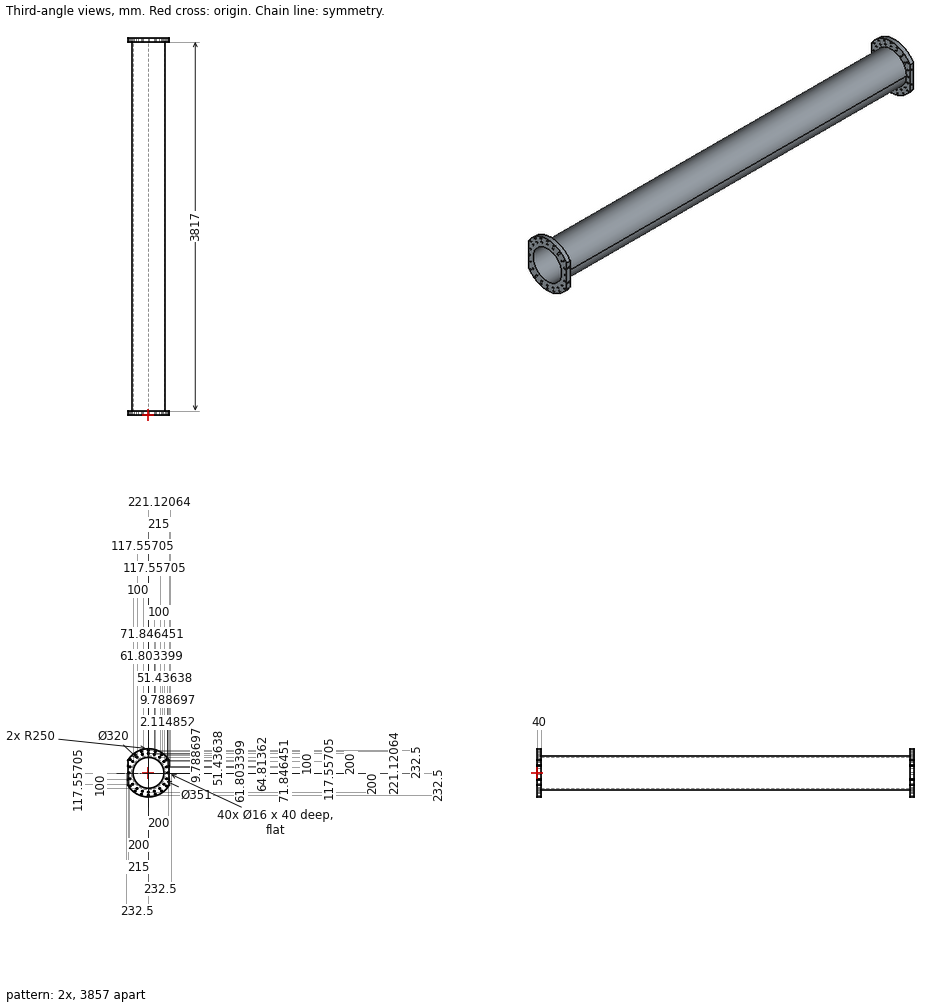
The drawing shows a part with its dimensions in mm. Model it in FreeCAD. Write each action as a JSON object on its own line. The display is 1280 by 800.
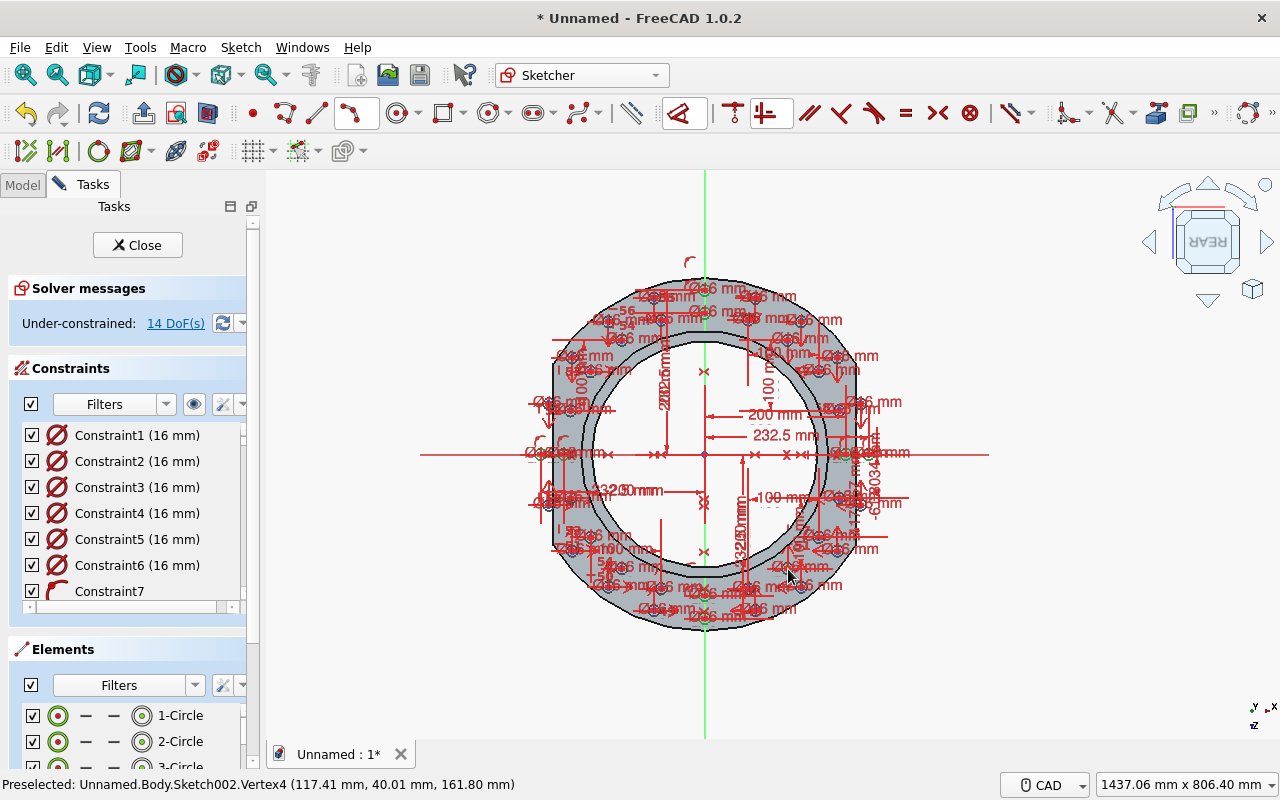
{"action": "key", "text": "l"}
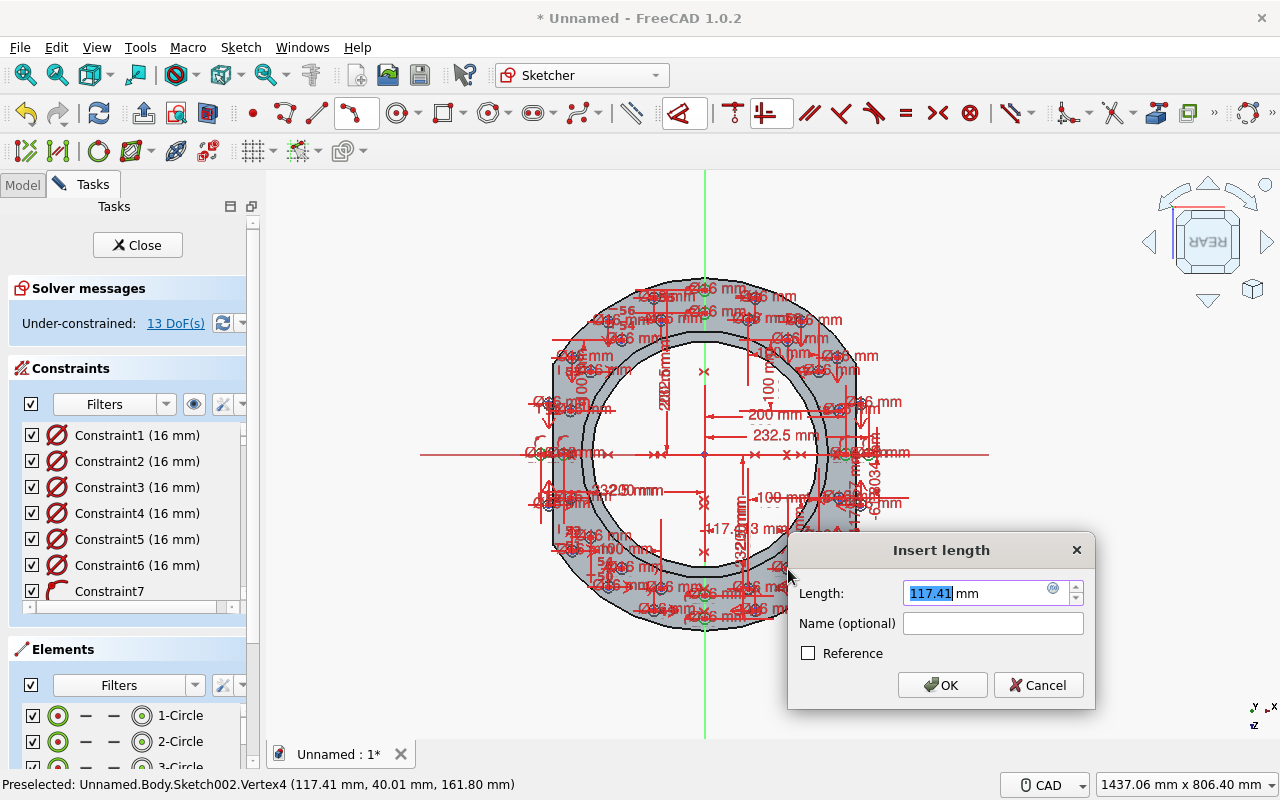
{"action": "type", "text": "117.55705"}
{"action": "key", "text": "Return"}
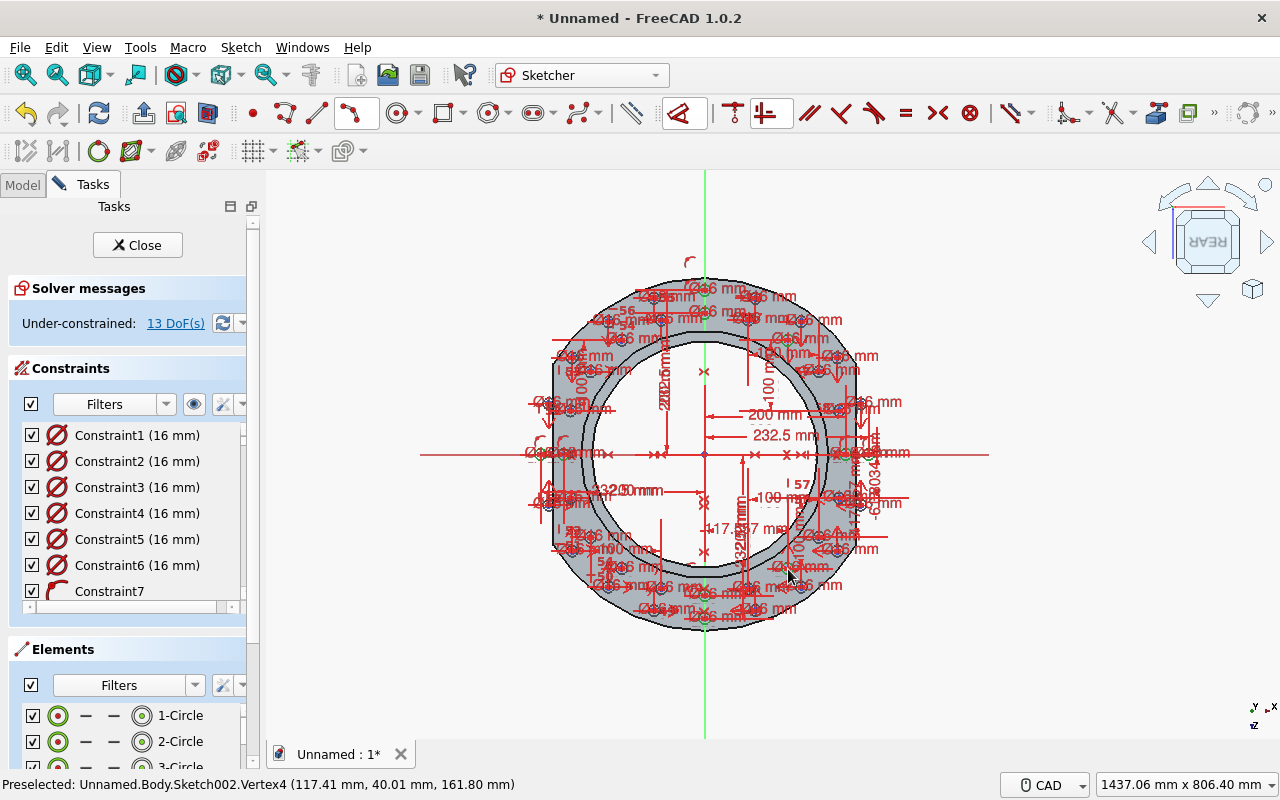
{"action": "left_click", "coordinate": [748, 589]}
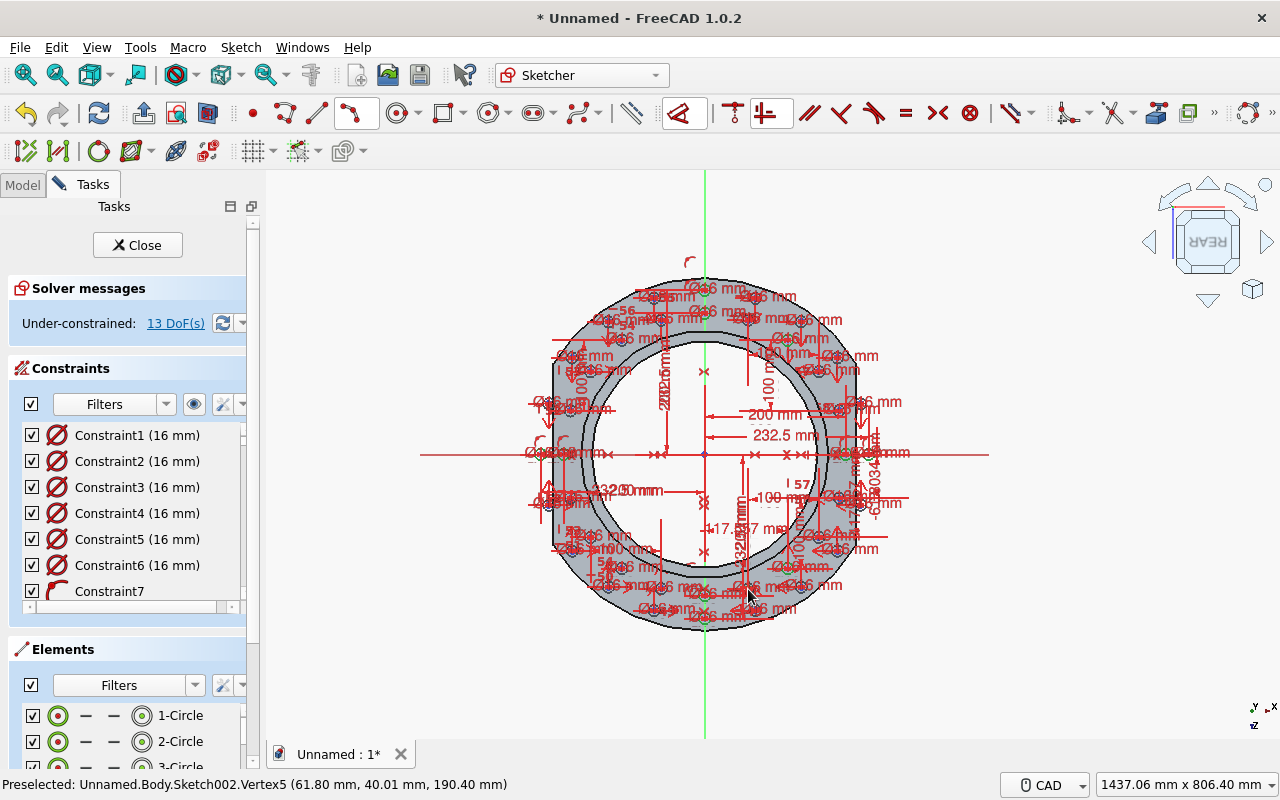
{"action": "key", "text": "l"}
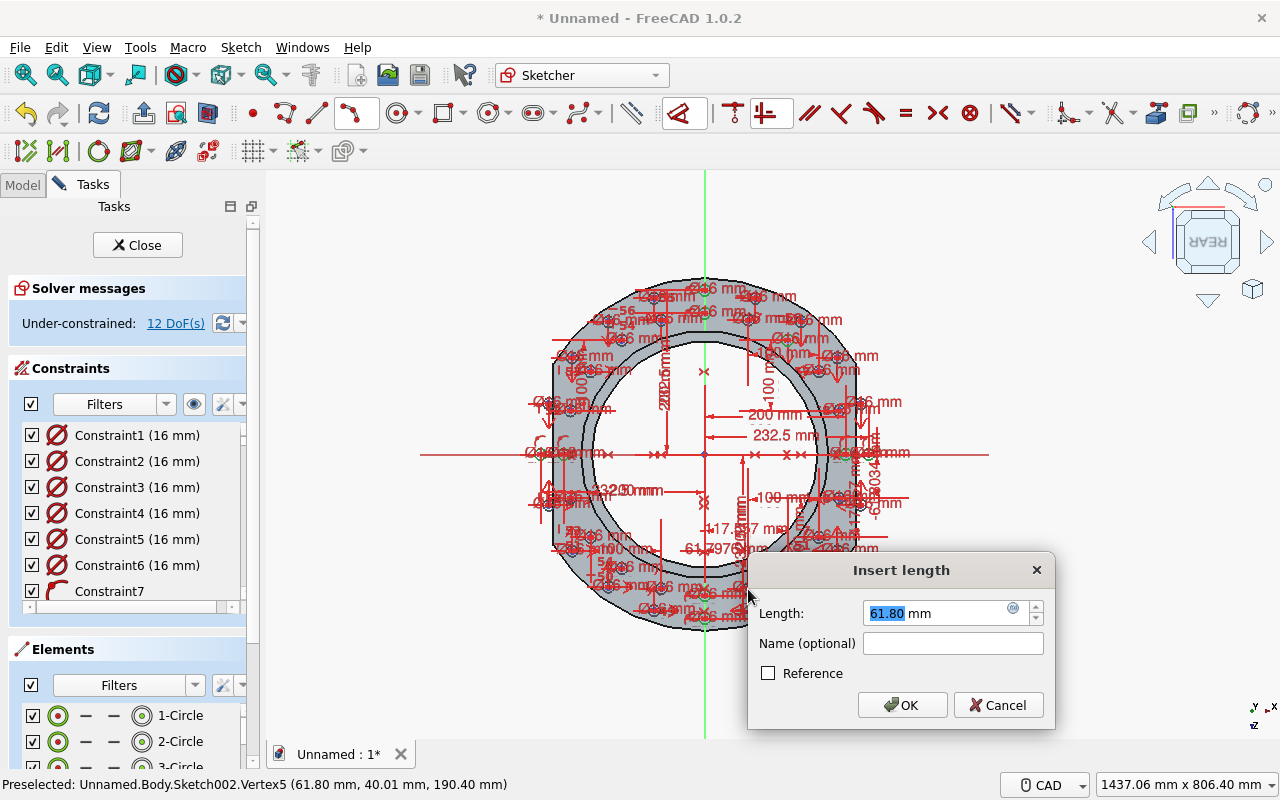
{"action": "type", "text": "61.803399"}
{"action": "key", "text": "Return"}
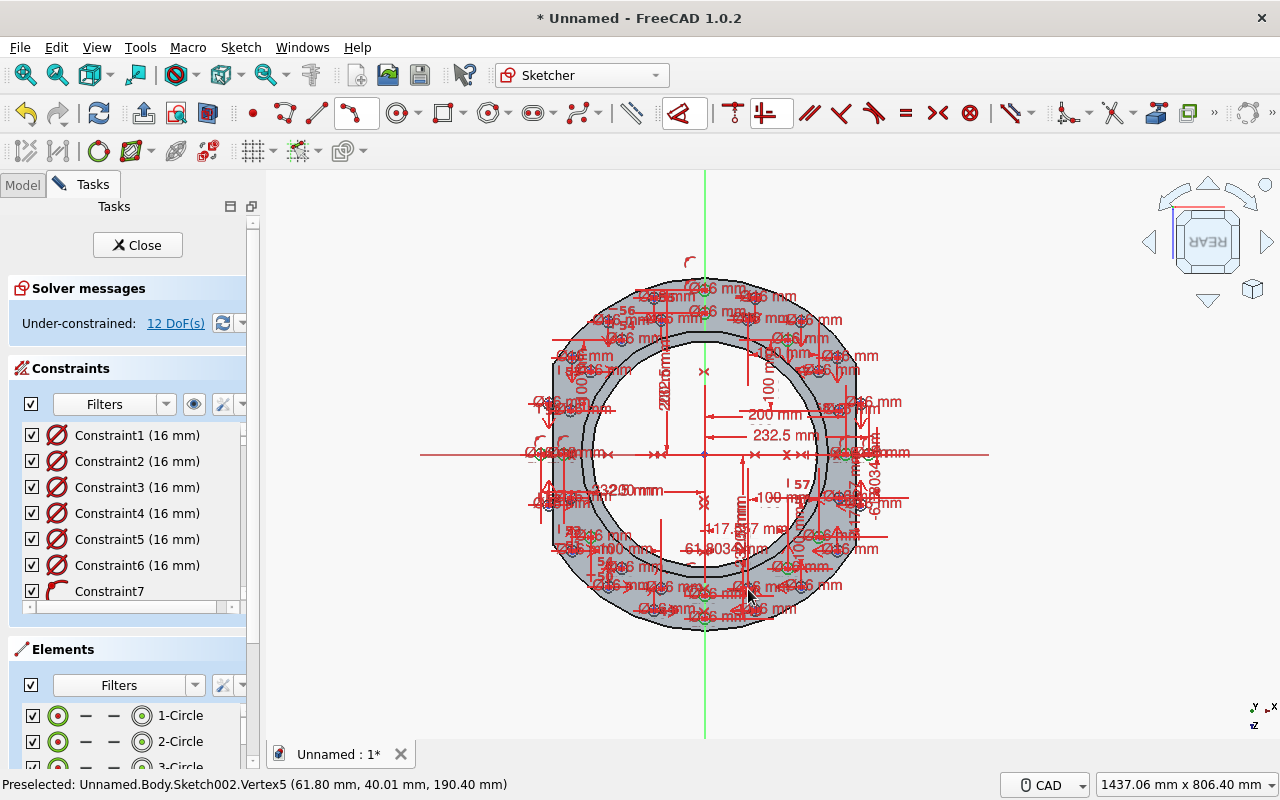
{"action": "left_click", "coordinate": [622, 569]}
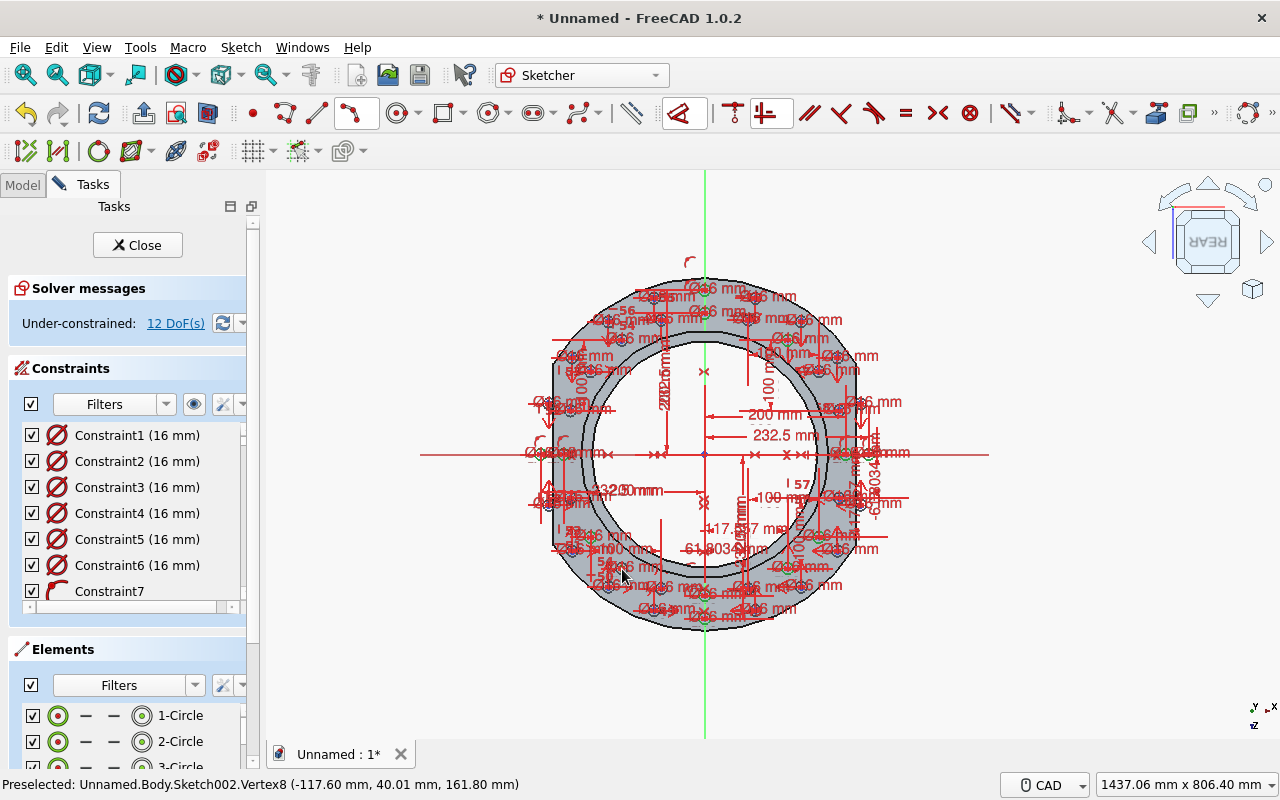
{"action": "key", "text": "l"}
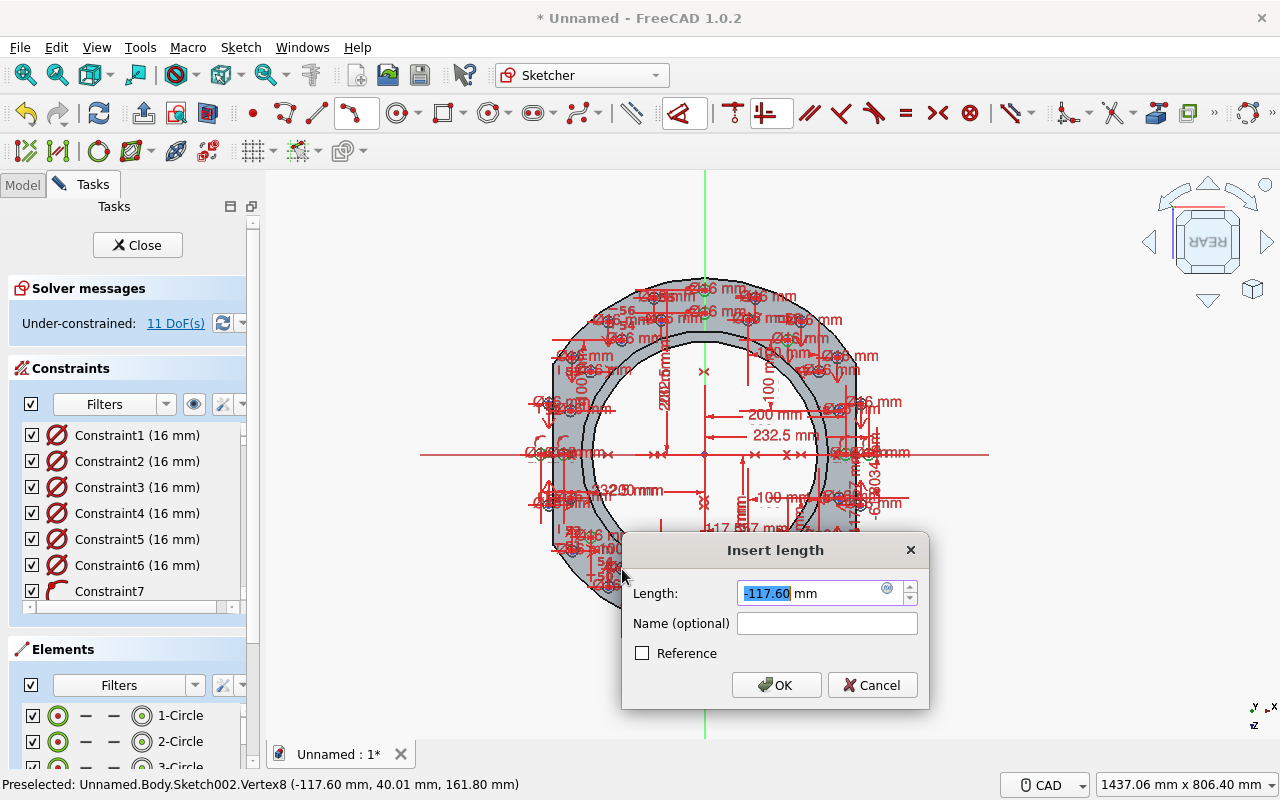
{"action": "type", "text": "-117.55705"}
{"action": "key", "text": "Return"}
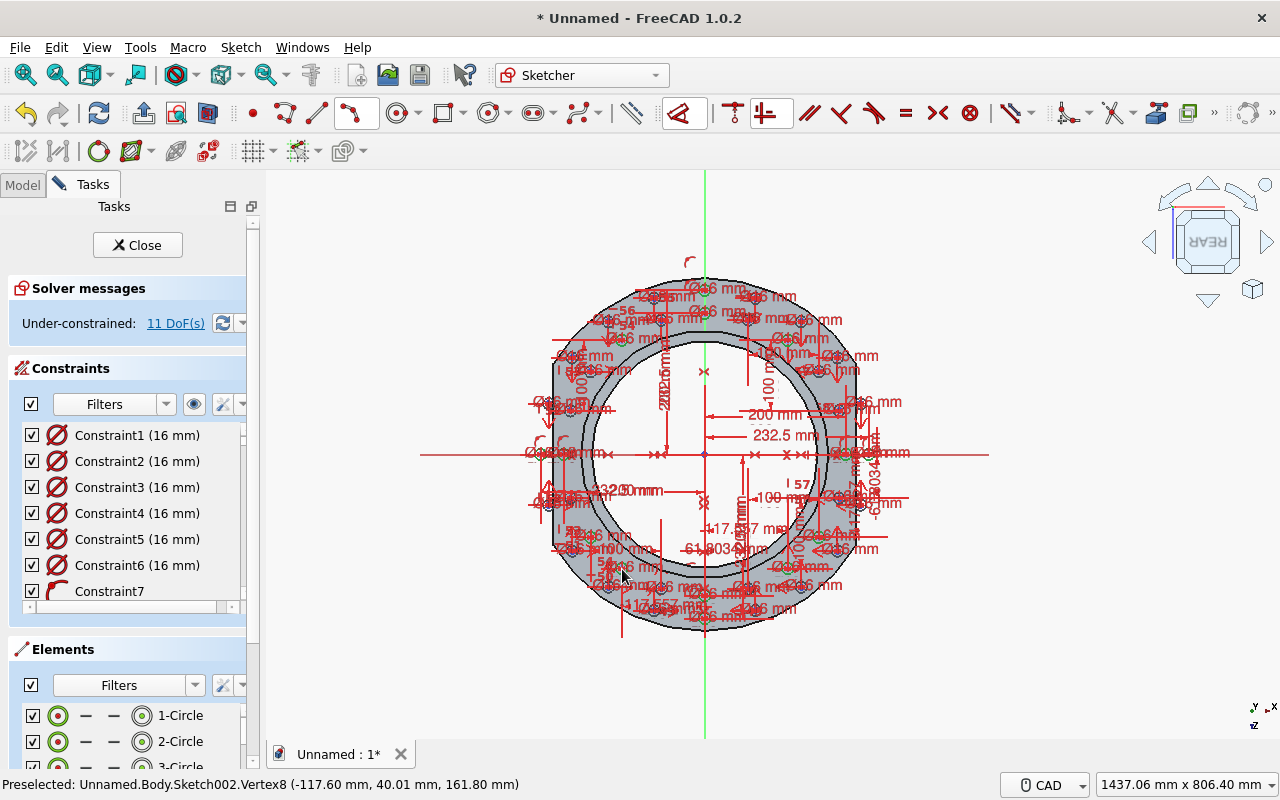
{"action": "left_click", "coordinate": [591, 372]}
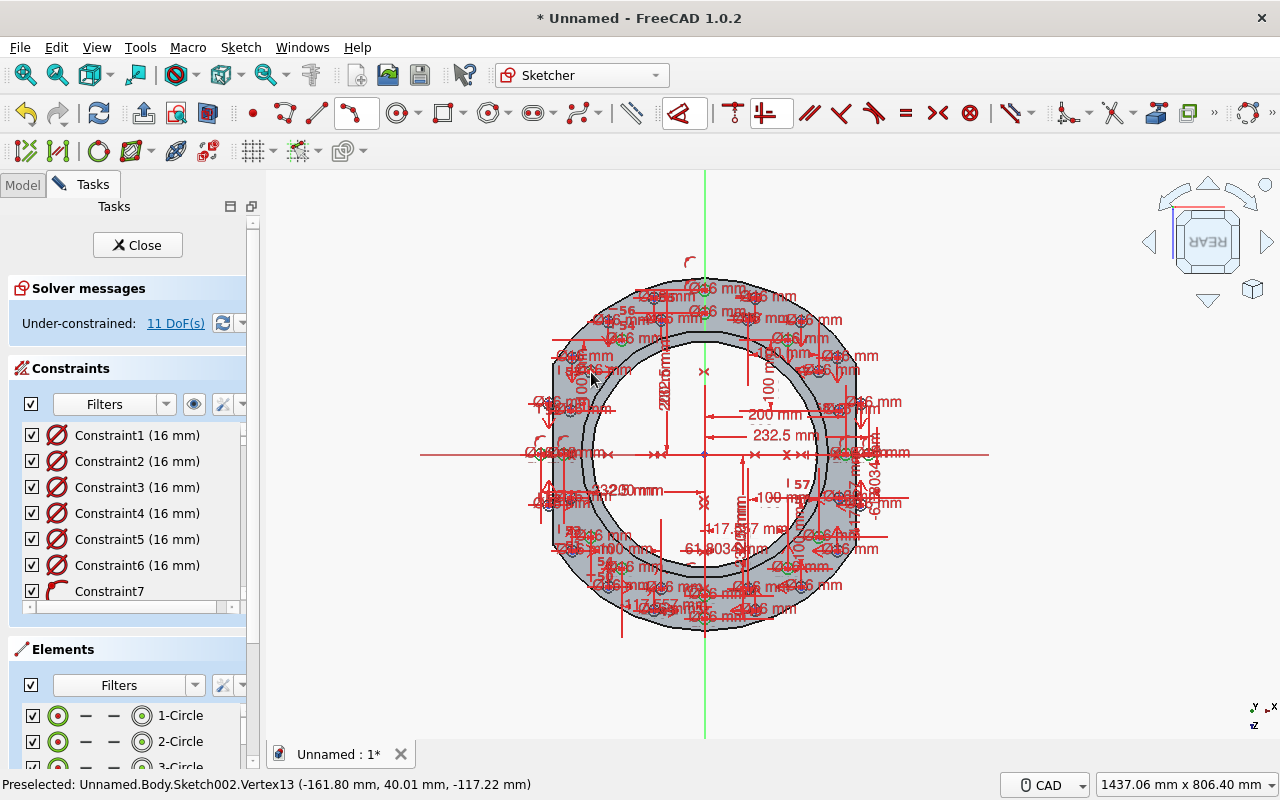
{"action": "left_click", "coordinate": [702, 114]}